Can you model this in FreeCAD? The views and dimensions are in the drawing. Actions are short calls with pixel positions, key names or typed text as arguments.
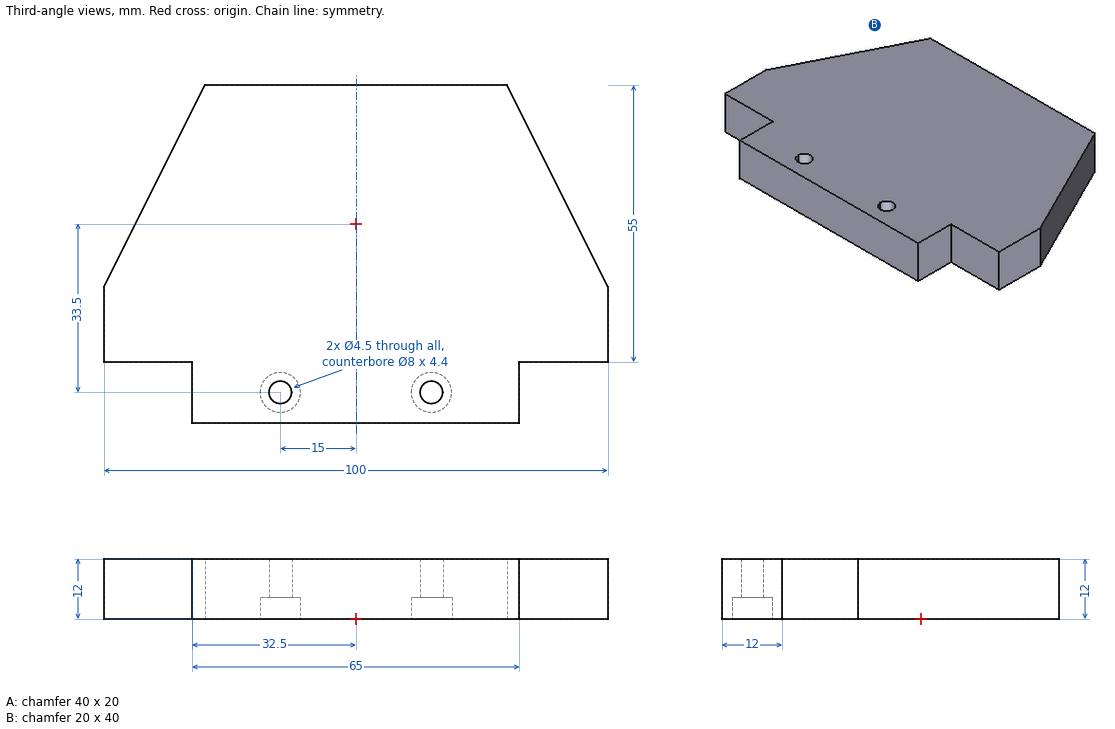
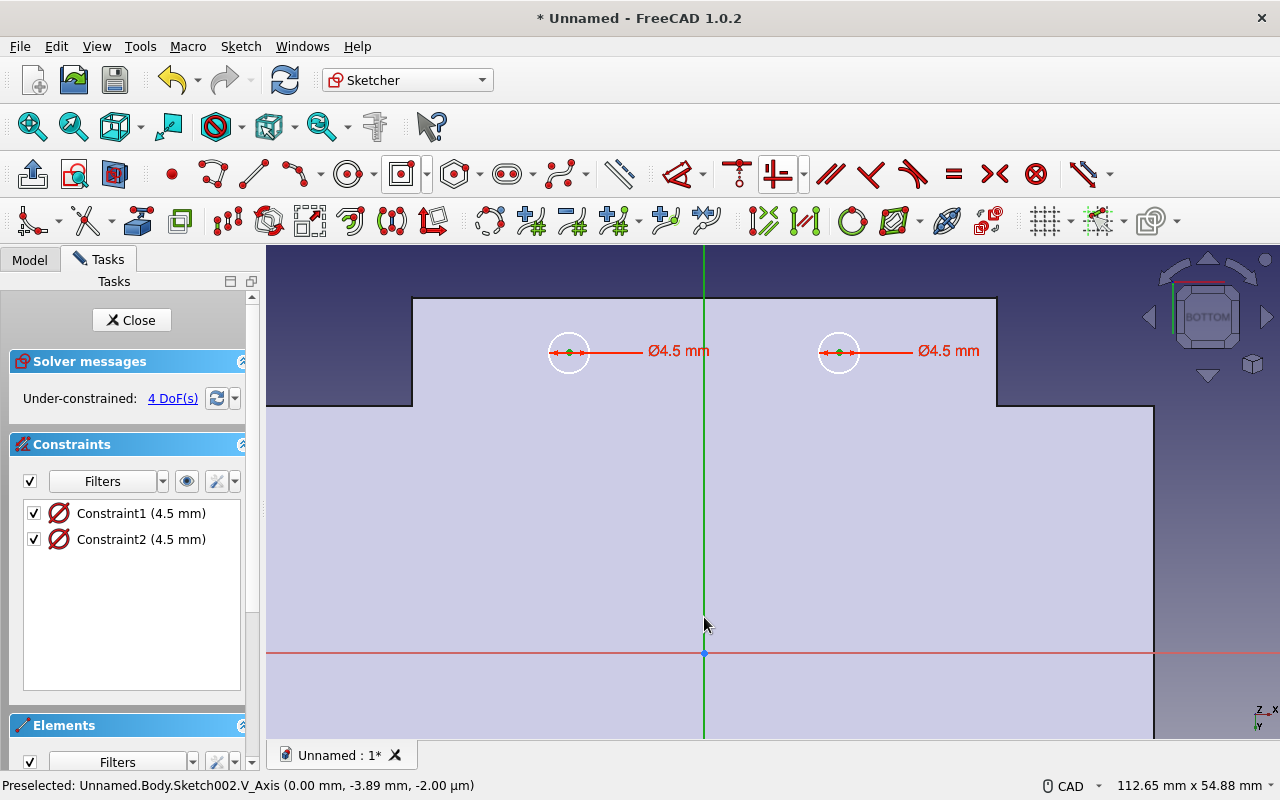
click(995, 174)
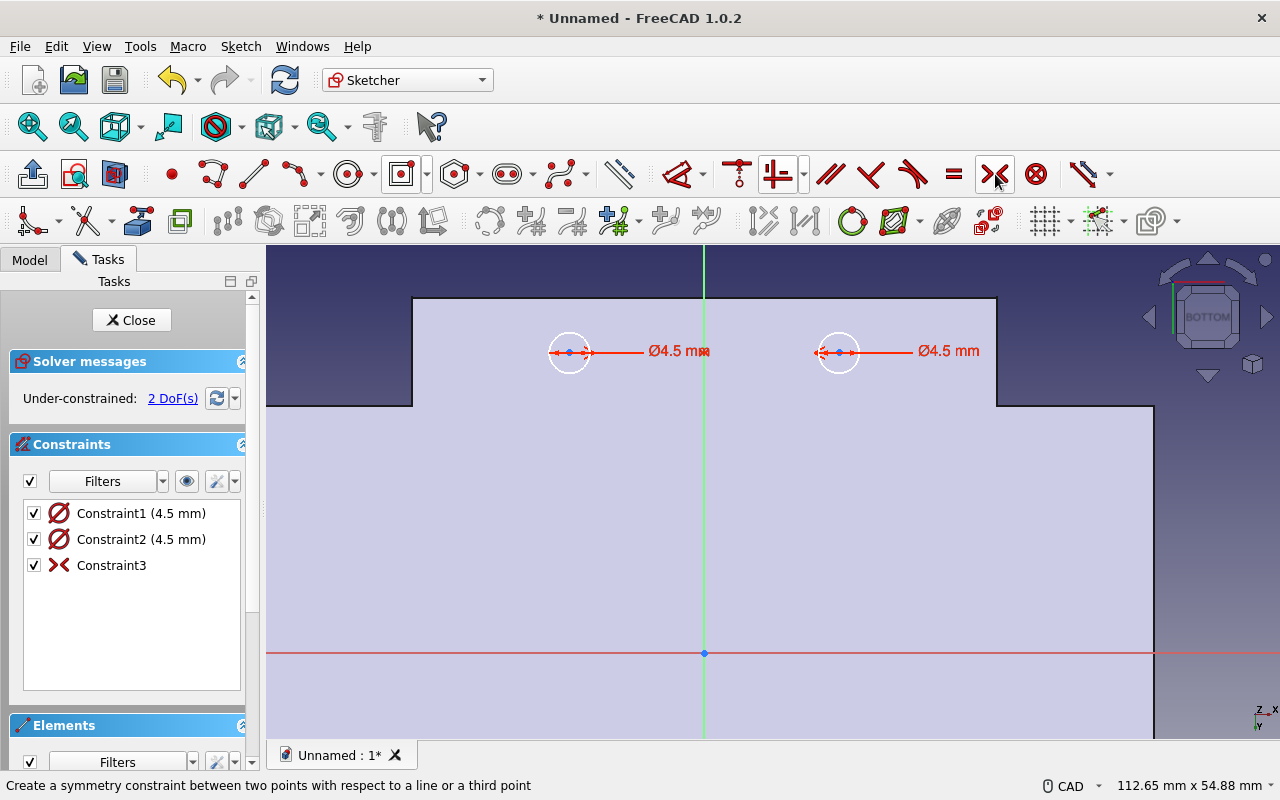
click(676, 174)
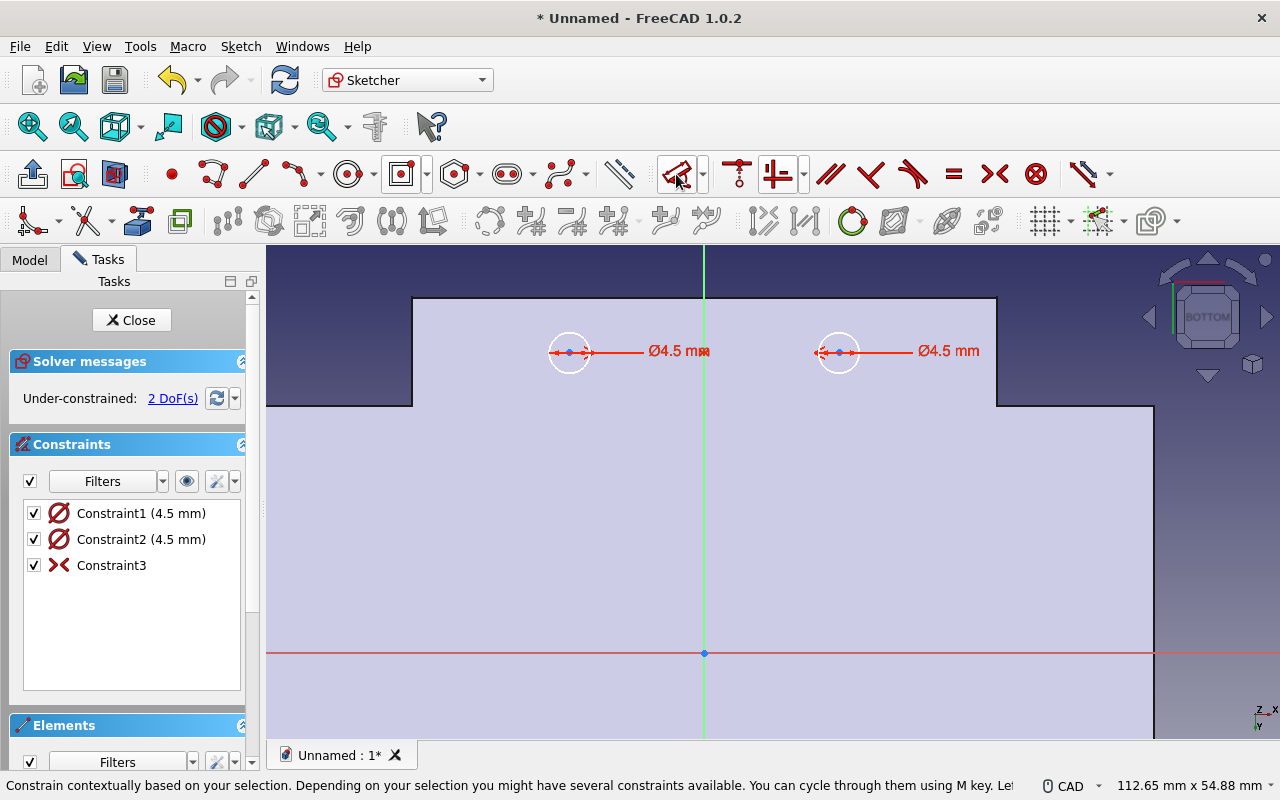
click(570, 353)
click(637, 687)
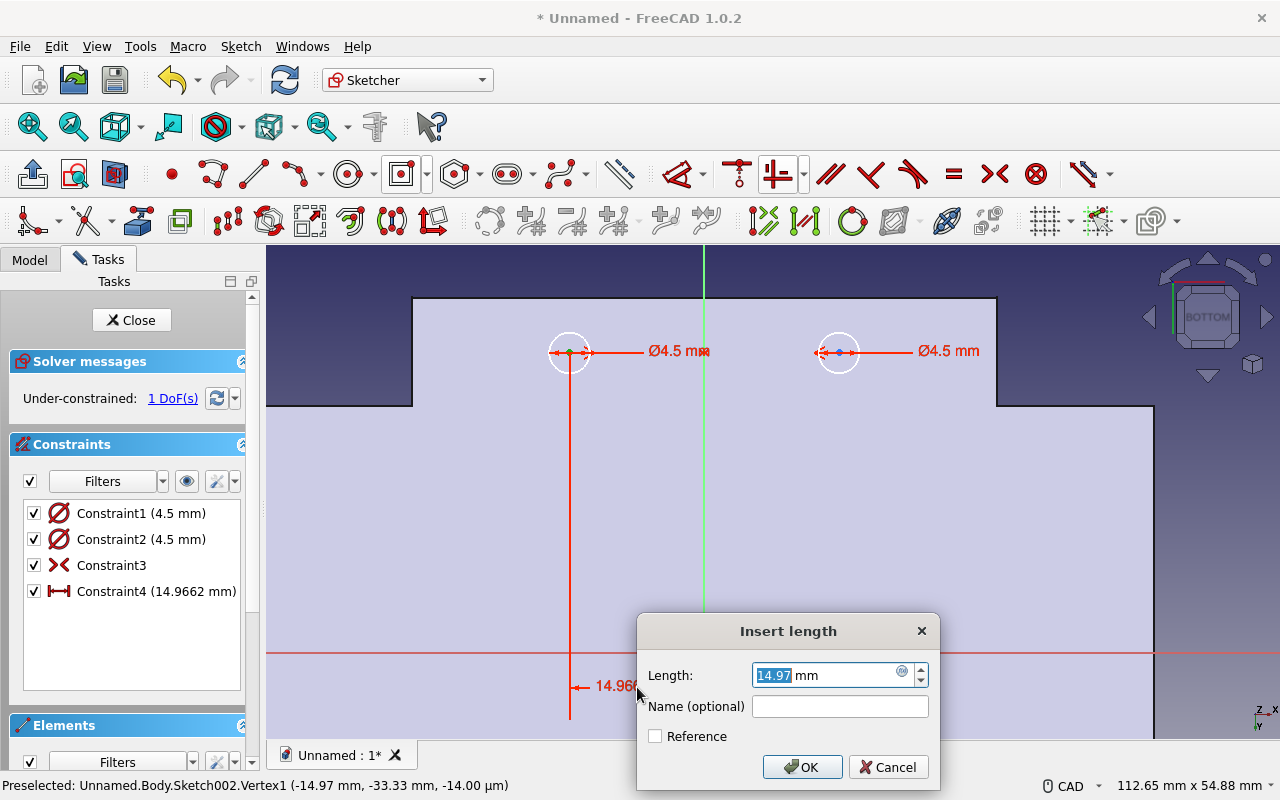
text(15)
key(Return)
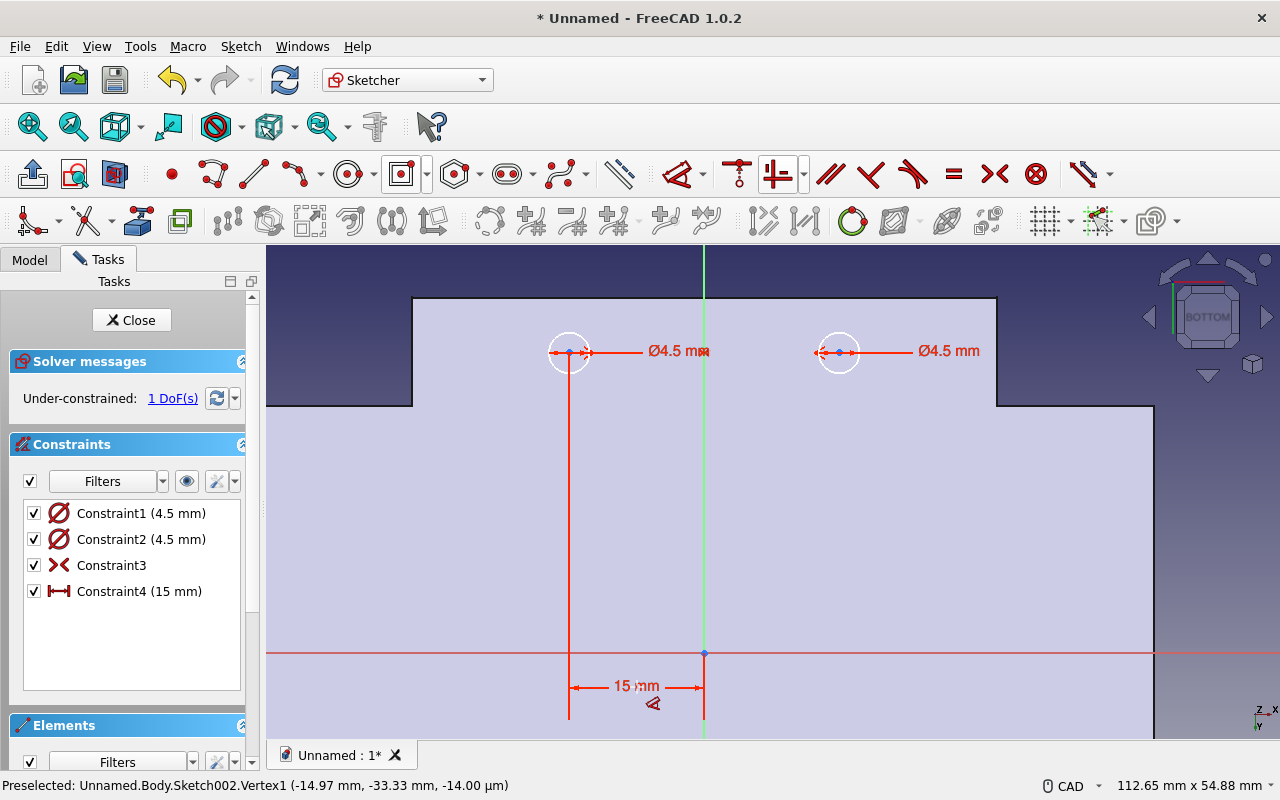
click(569, 353)
click(535, 503)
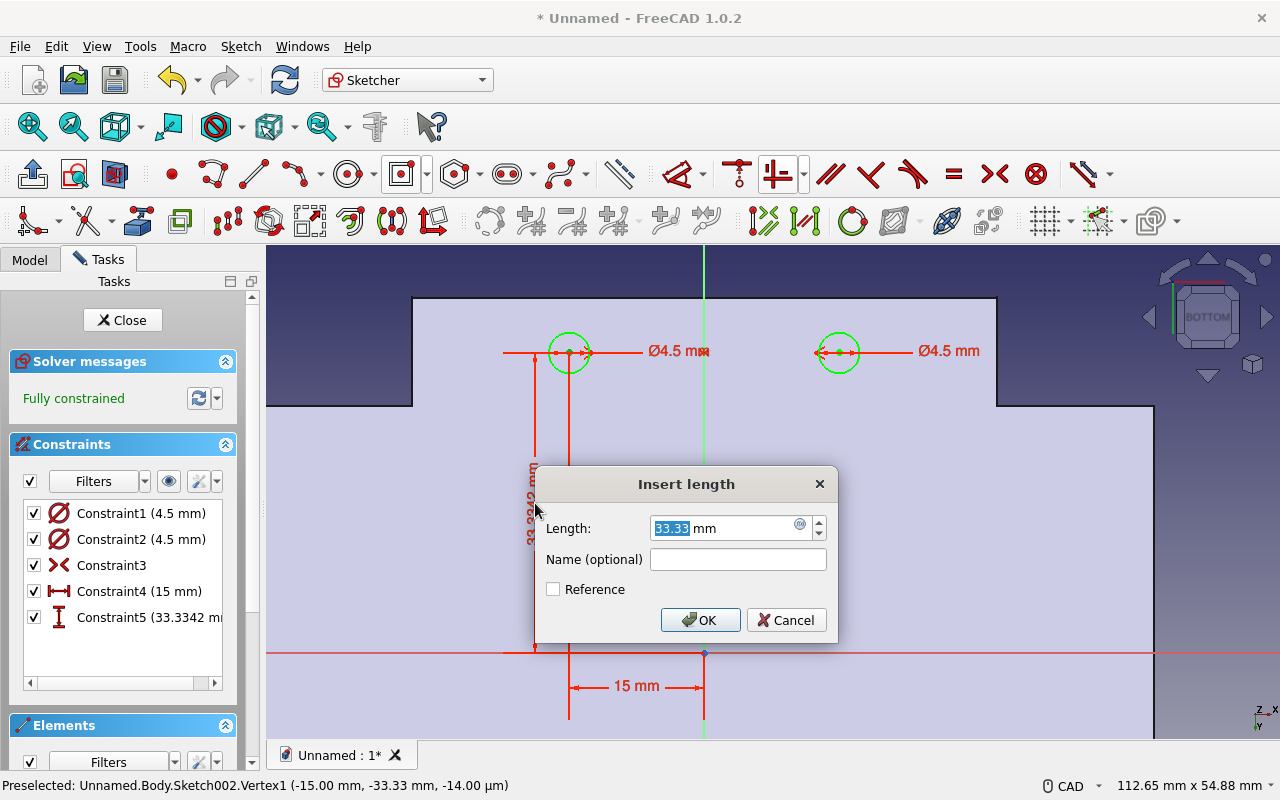
text(33.5)
key(Return)
key(Escape)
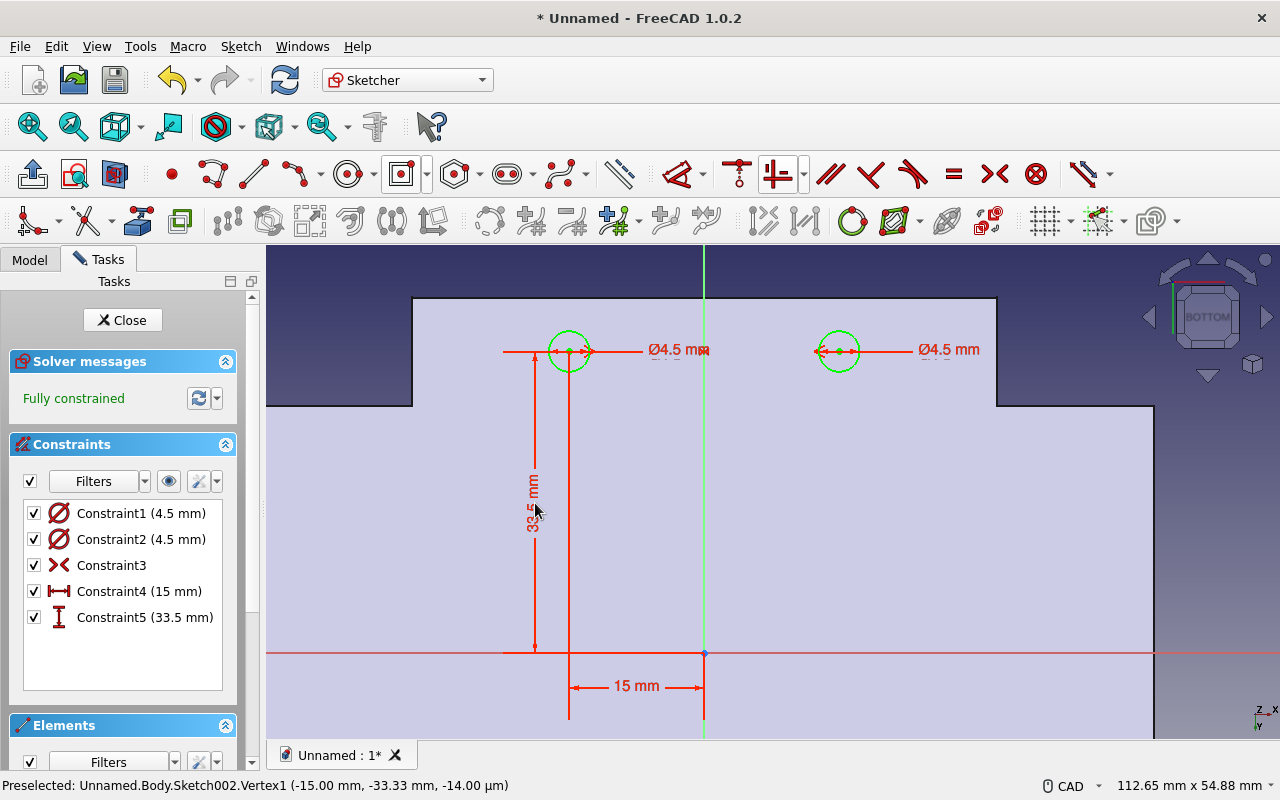
click(123, 320)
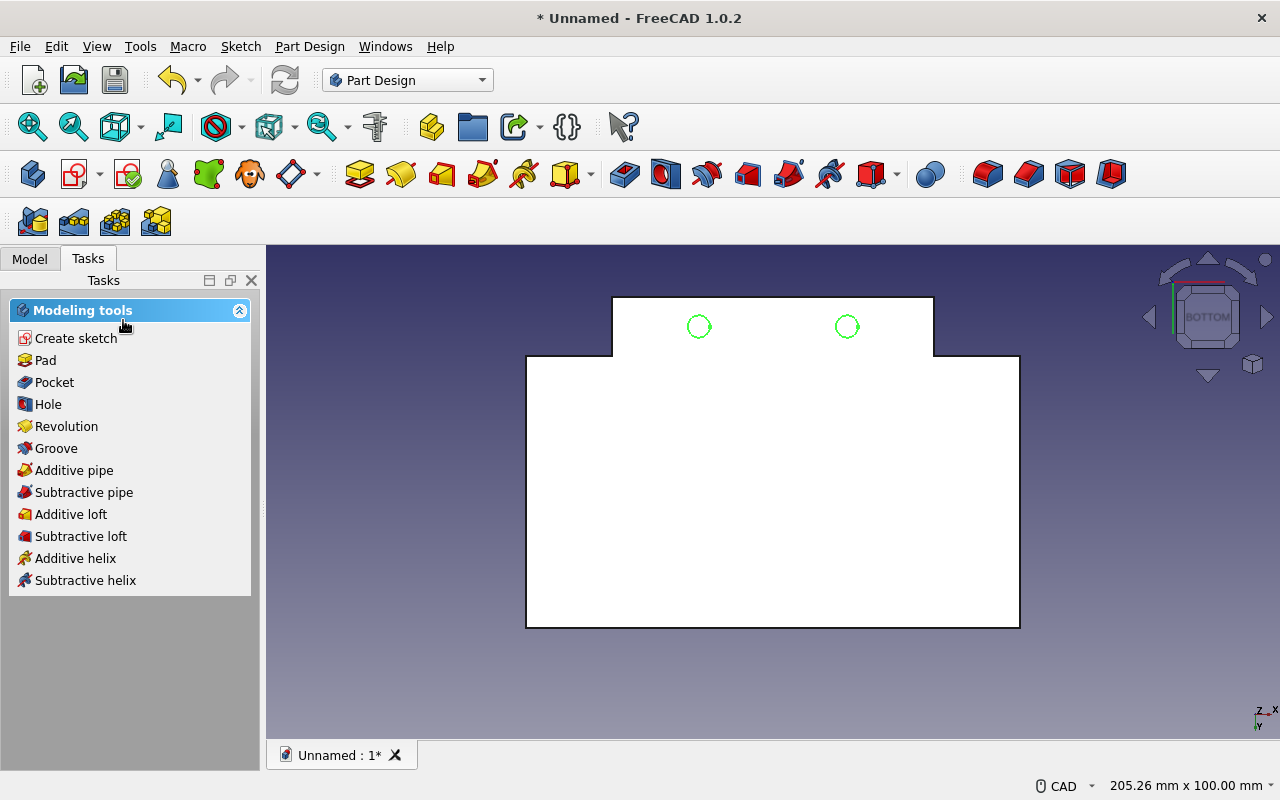
click(666, 174)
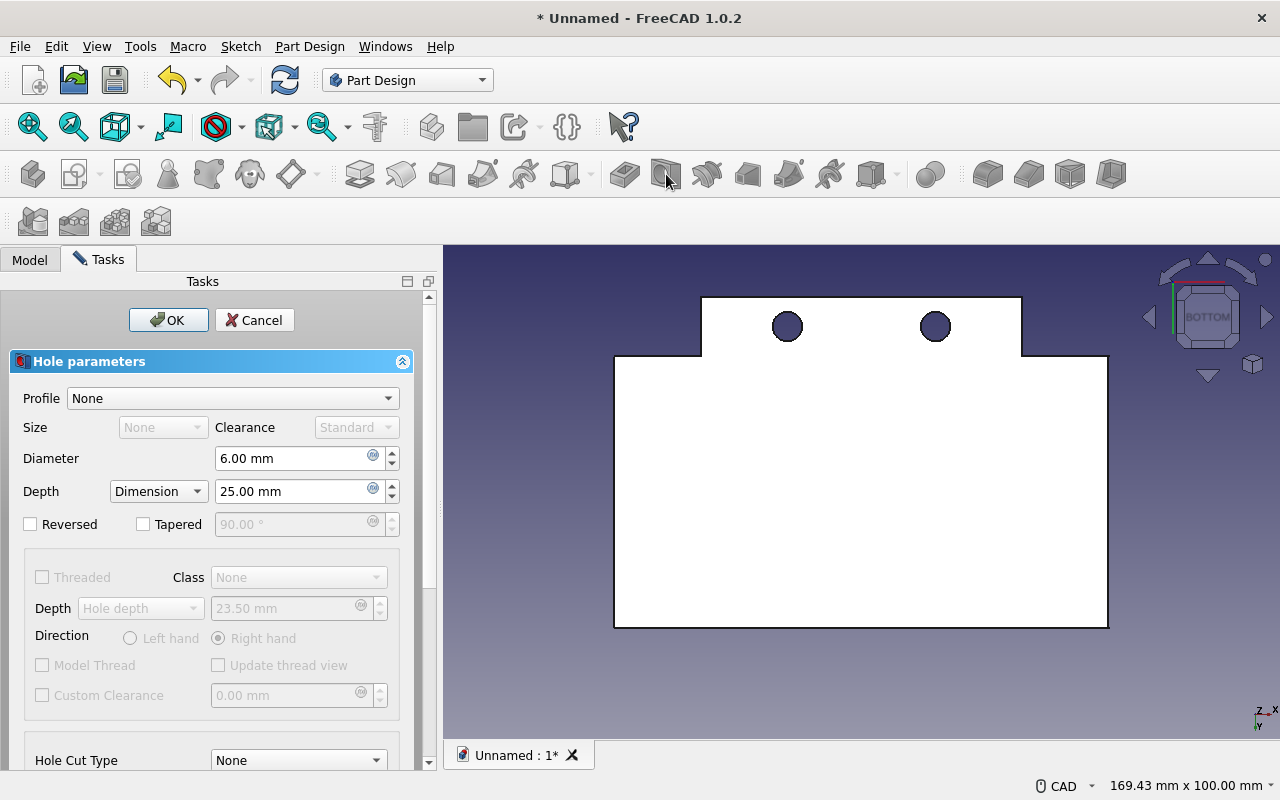
triple_click(300, 458)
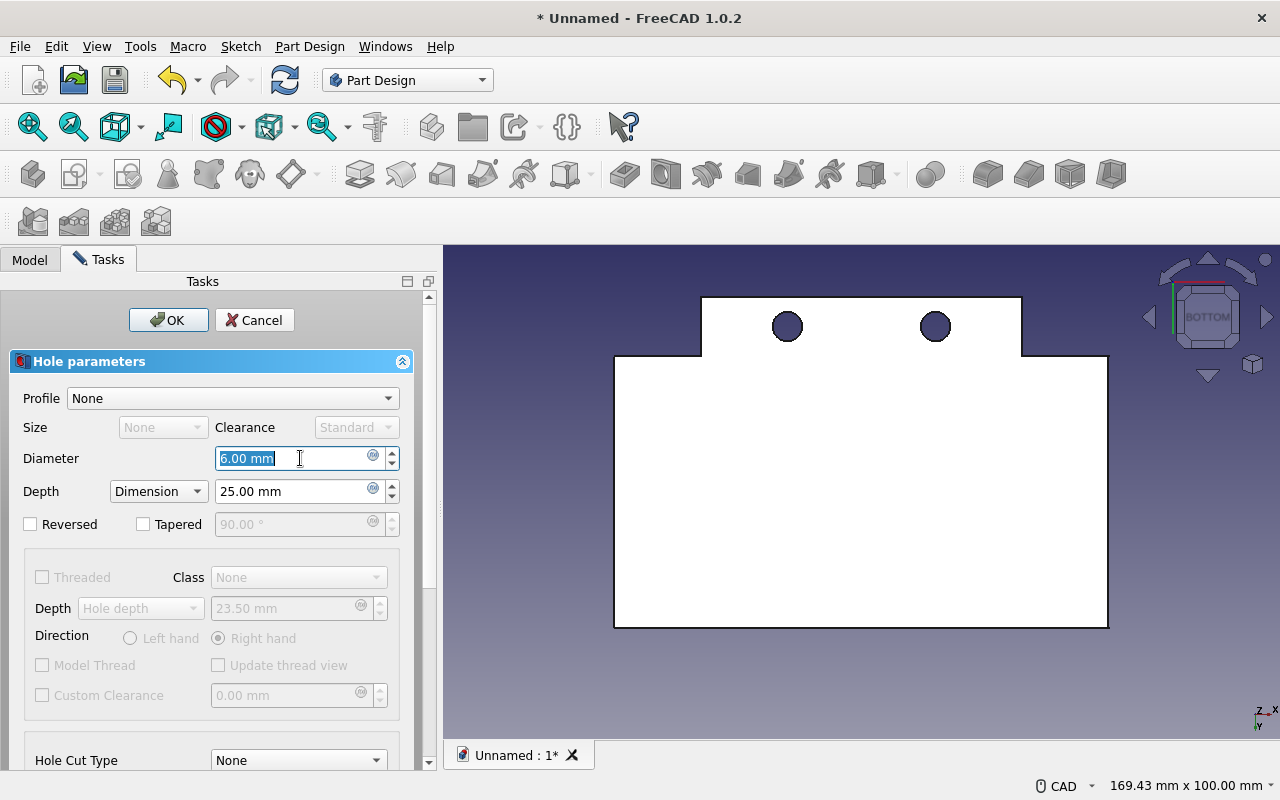
text(4.5)
key(Tab)